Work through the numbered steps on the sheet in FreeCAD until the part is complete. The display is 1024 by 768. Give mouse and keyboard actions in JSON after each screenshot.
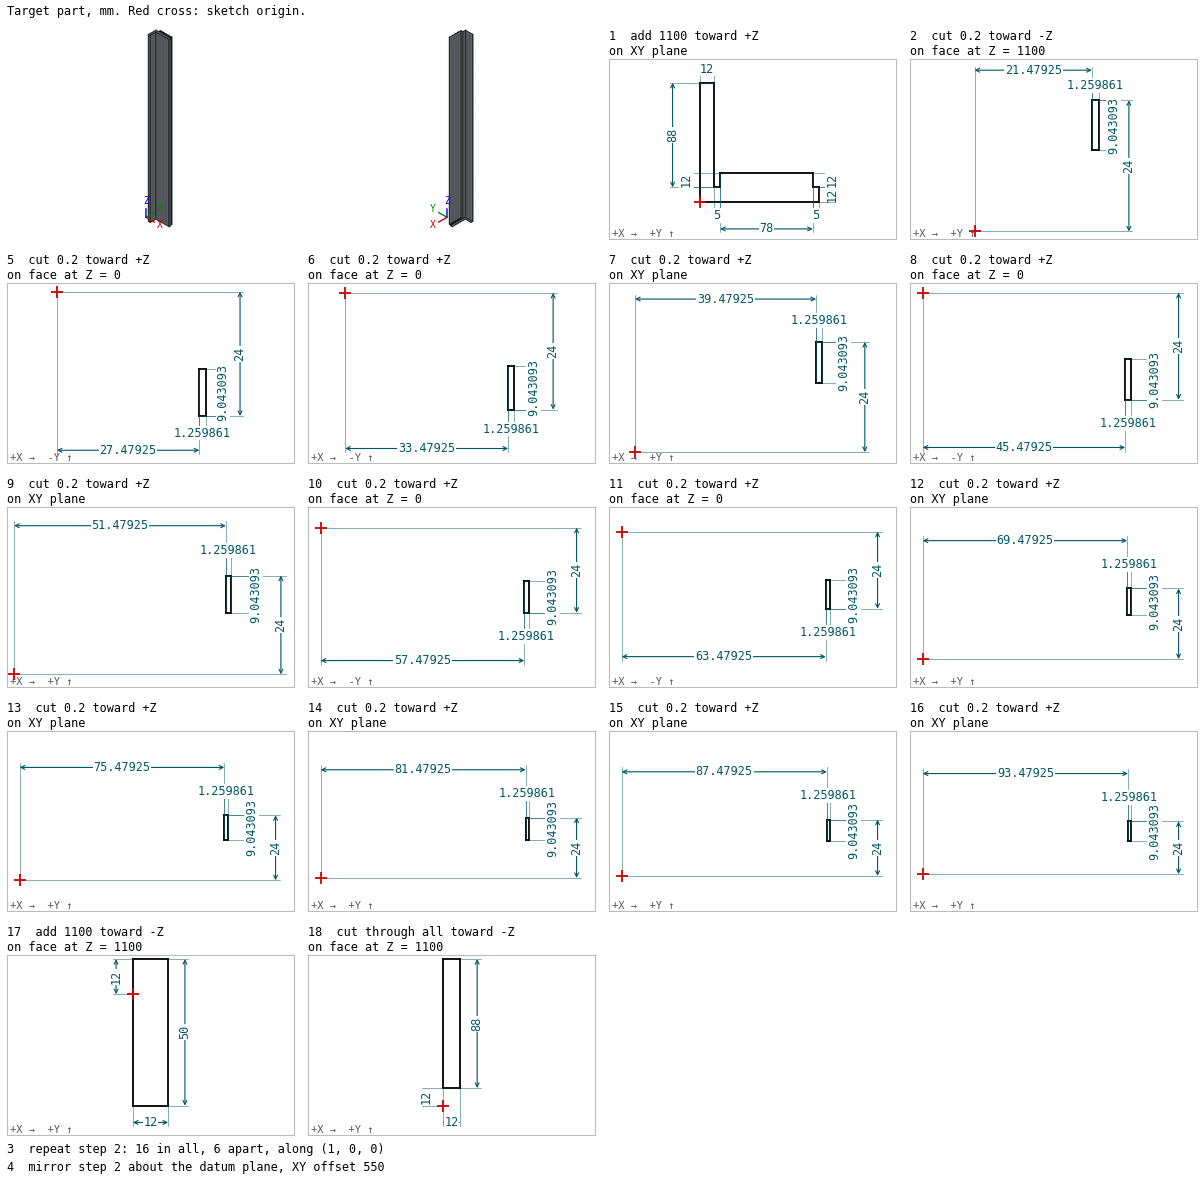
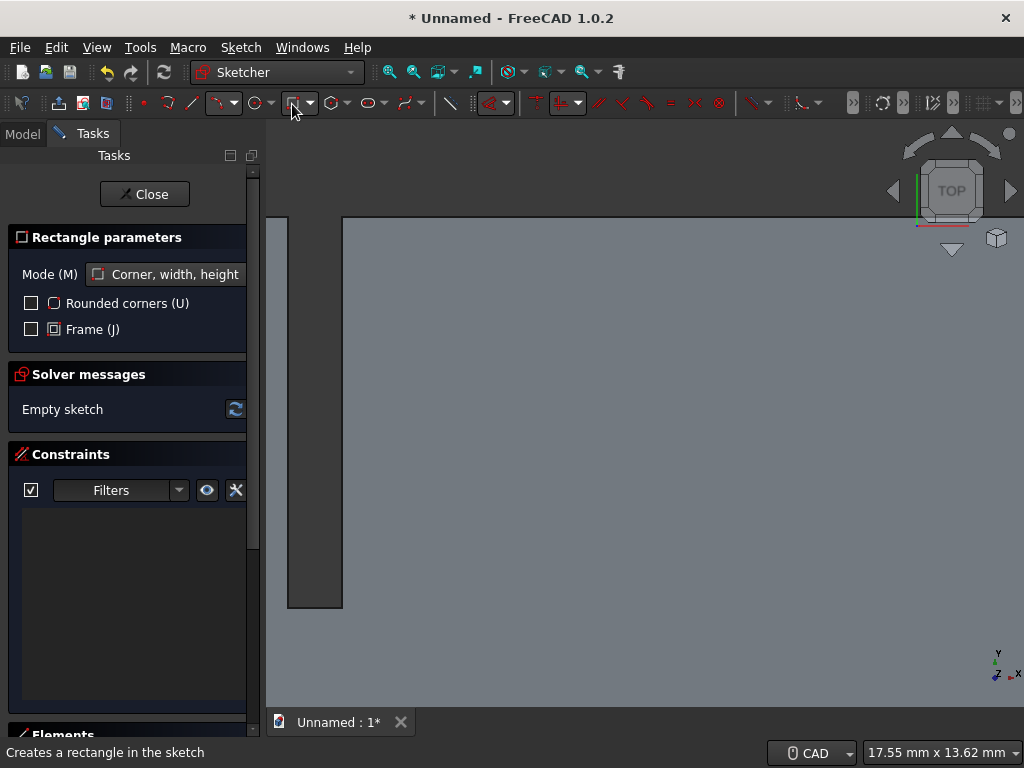
{"action": "left_click", "coordinate": [547, 217]}
{"action": "mouse_move", "coordinate": [601, 608]}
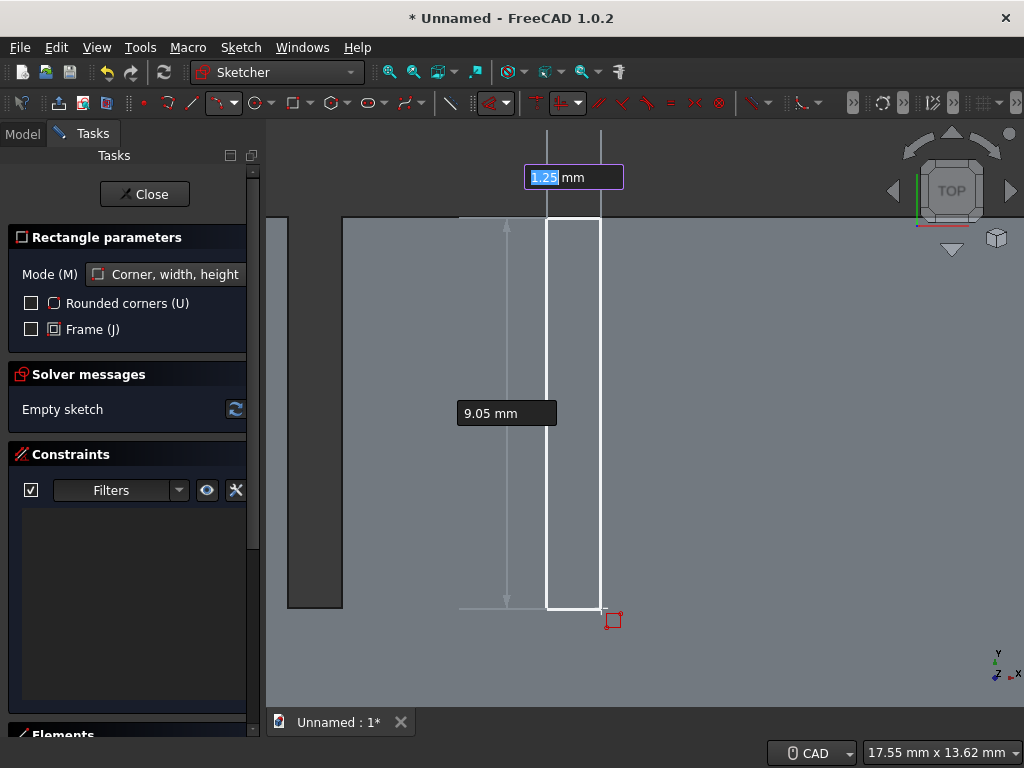
{"action": "type", "text": "1.259861"}
{"action": "key", "text": "Tab"}
{"action": "type", "text": "9.043093"}
{"action": "key", "text": "Return"}
{"action": "key", "text": "Escape"}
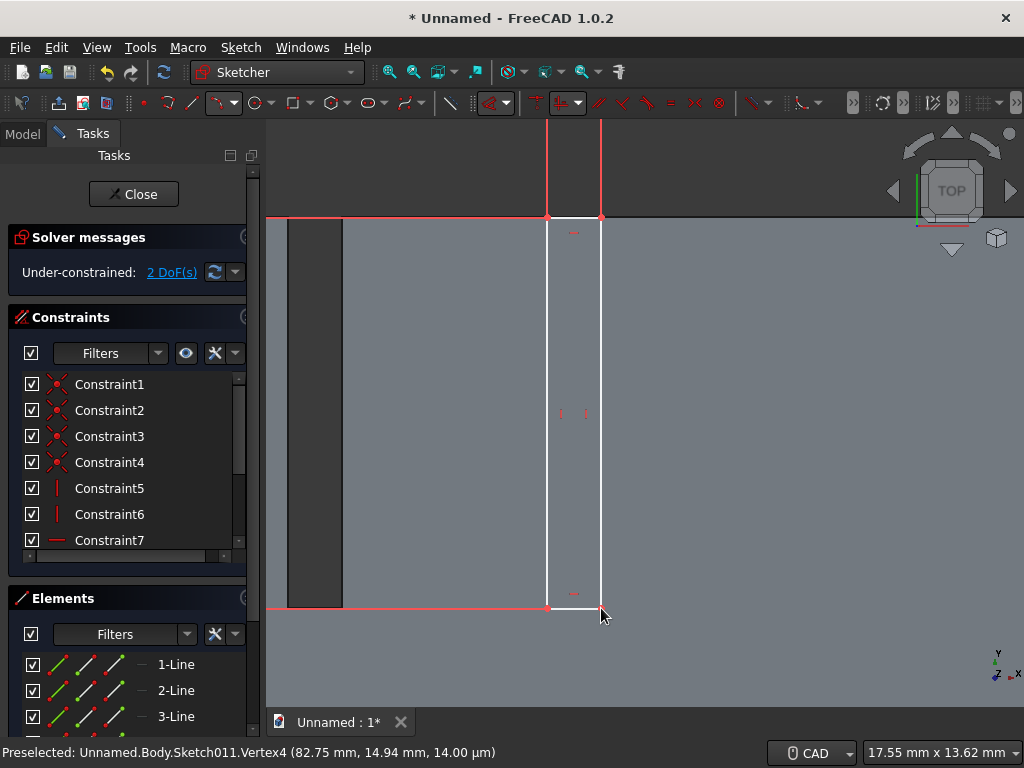
{"action": "left_click", "coordinate": [547, 218]}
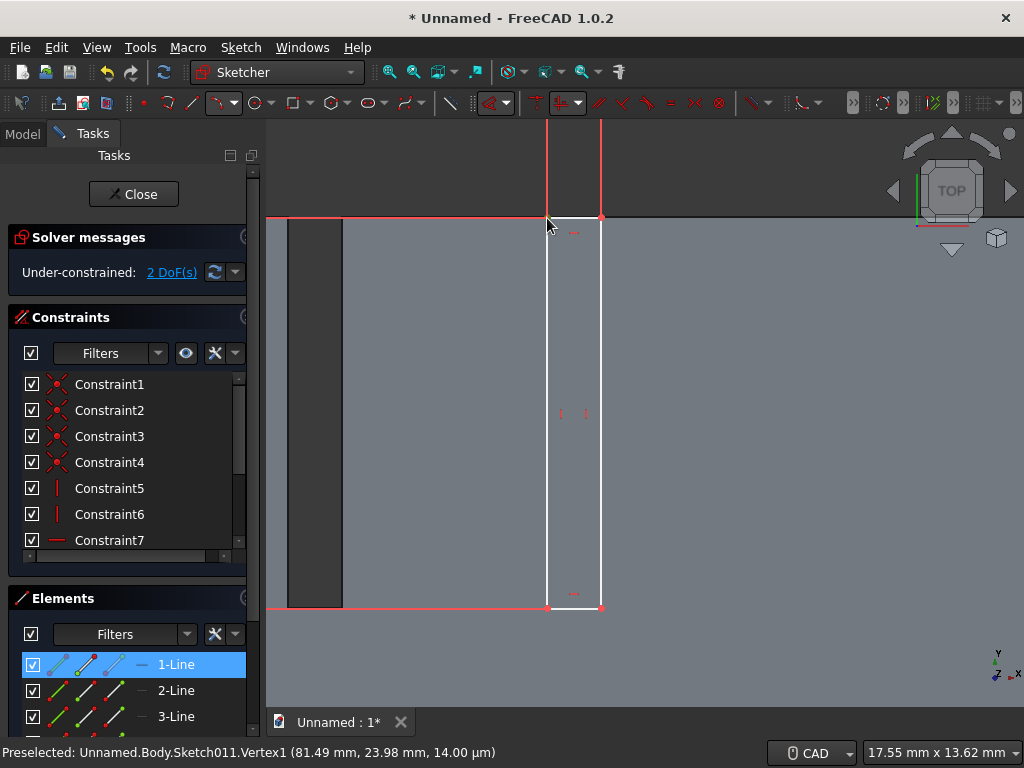
{"action": "left_click", "coordinate": [508, 104]}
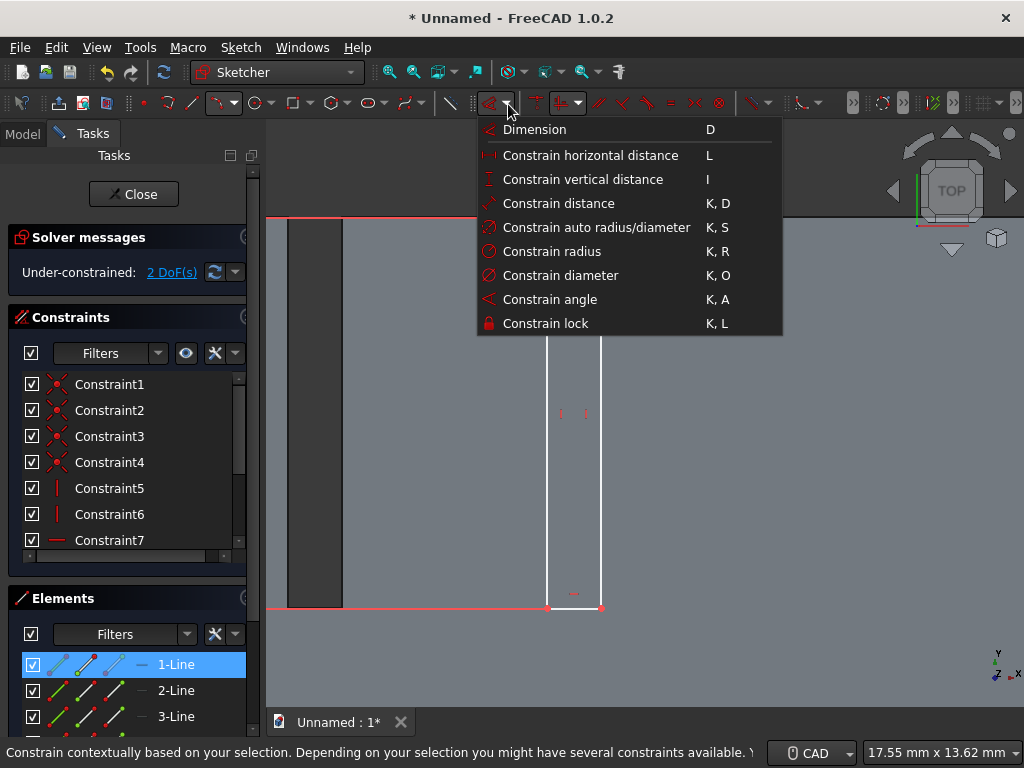
{"action": "left_click", "coordinate": [630, 179]}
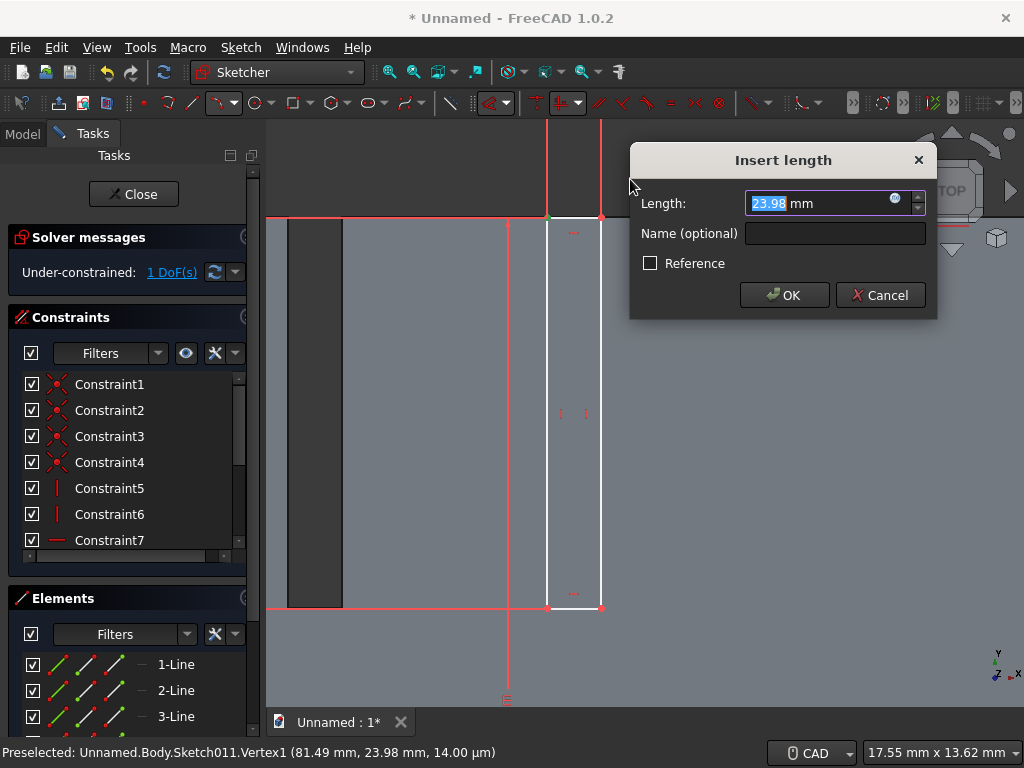
{"action": "type", "text": "24"}
{"action": "key", "text": "Return"}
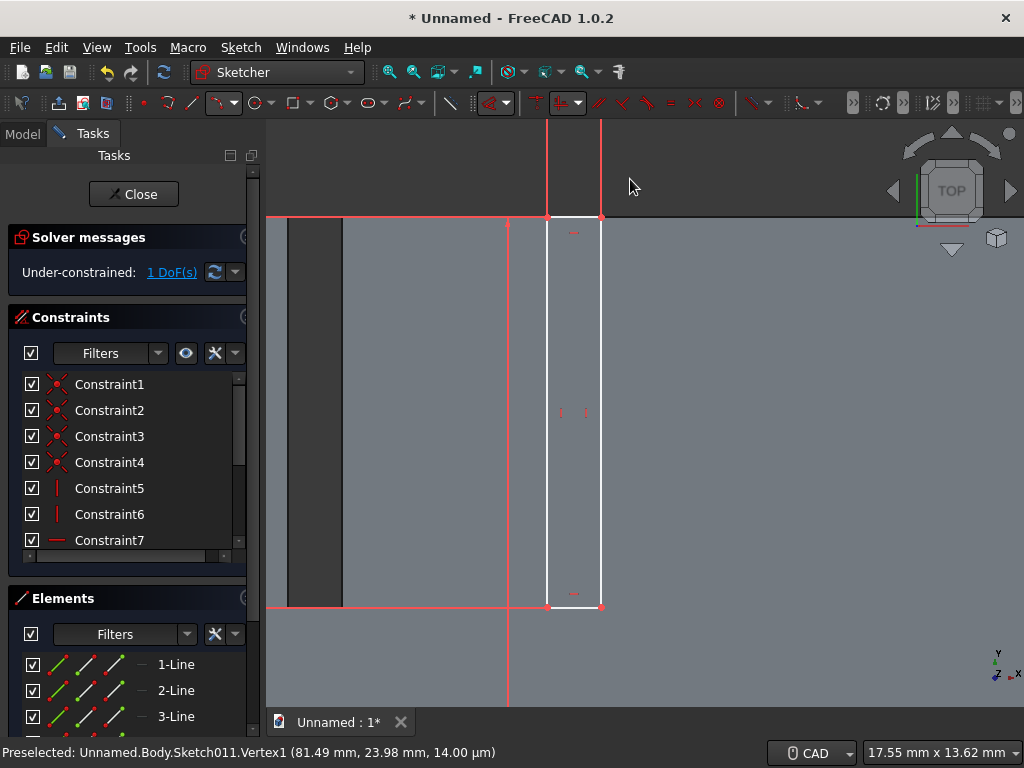
{"action": "left_click", "coordinate": [547, 217]}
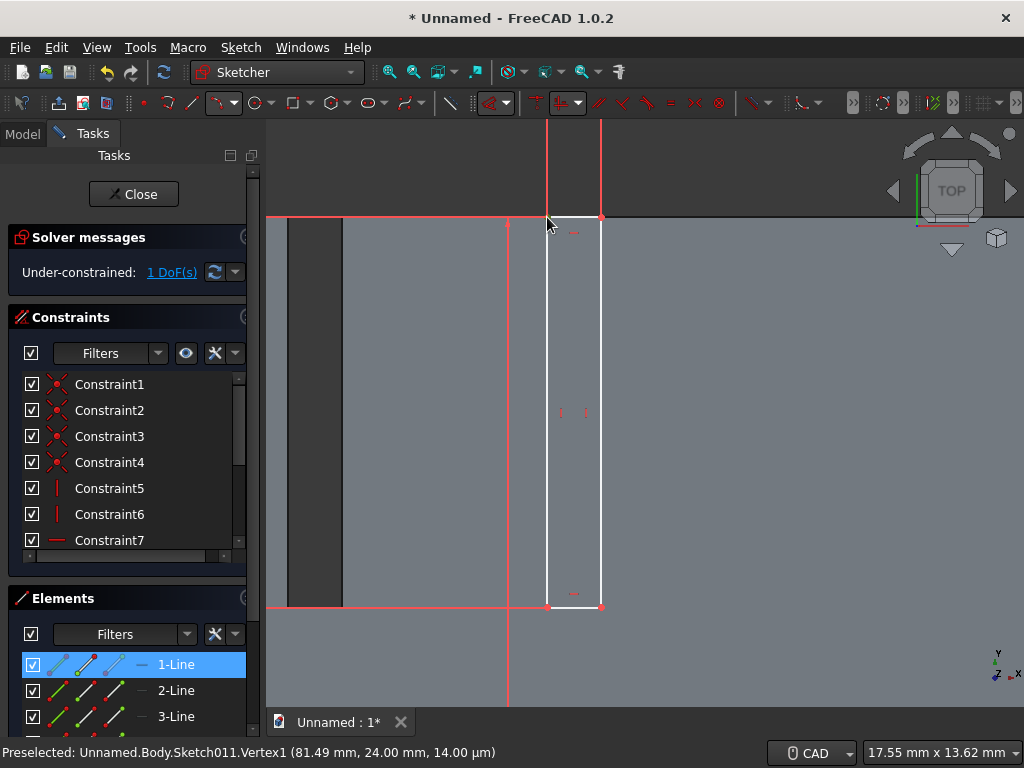
{"action": "key", "text": "l"}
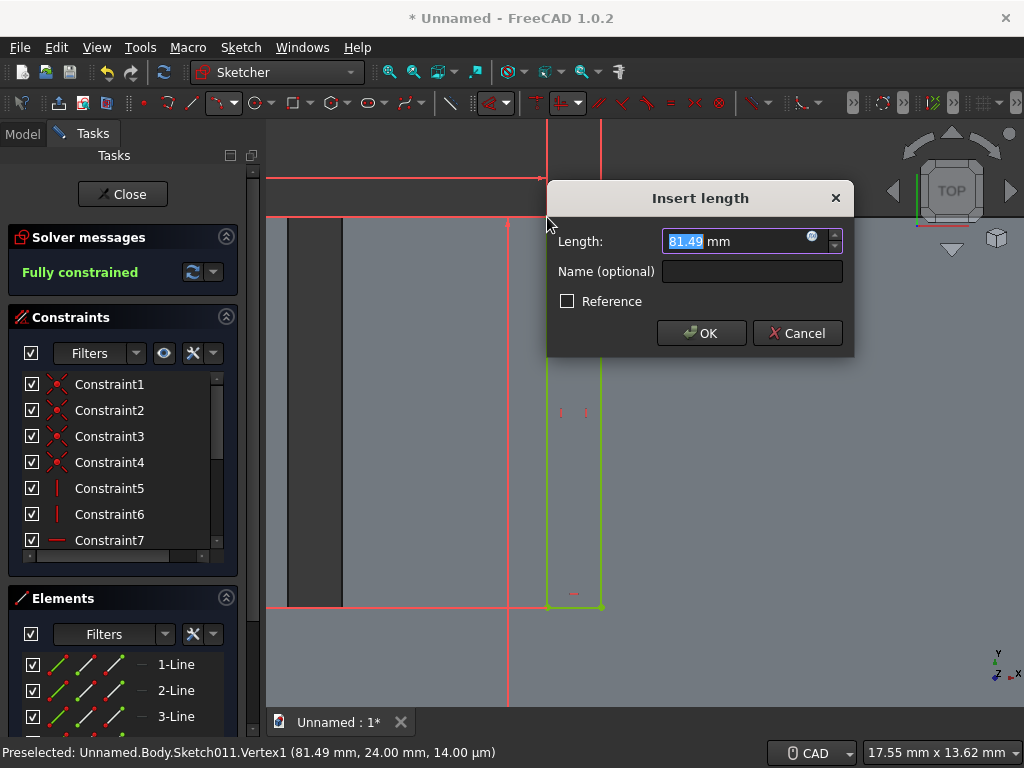
{"action": "type", "text": "81.47925"}
{"action": "key", "text": "Return"}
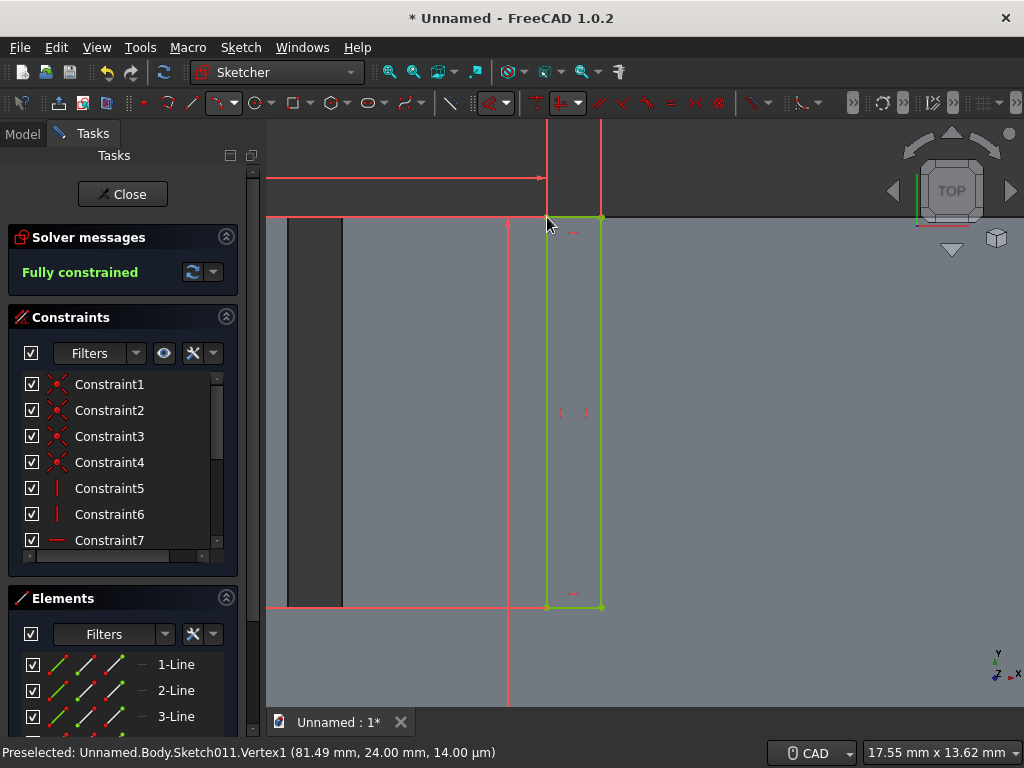
{"action": "left_click", "coordinate": [123, 194]}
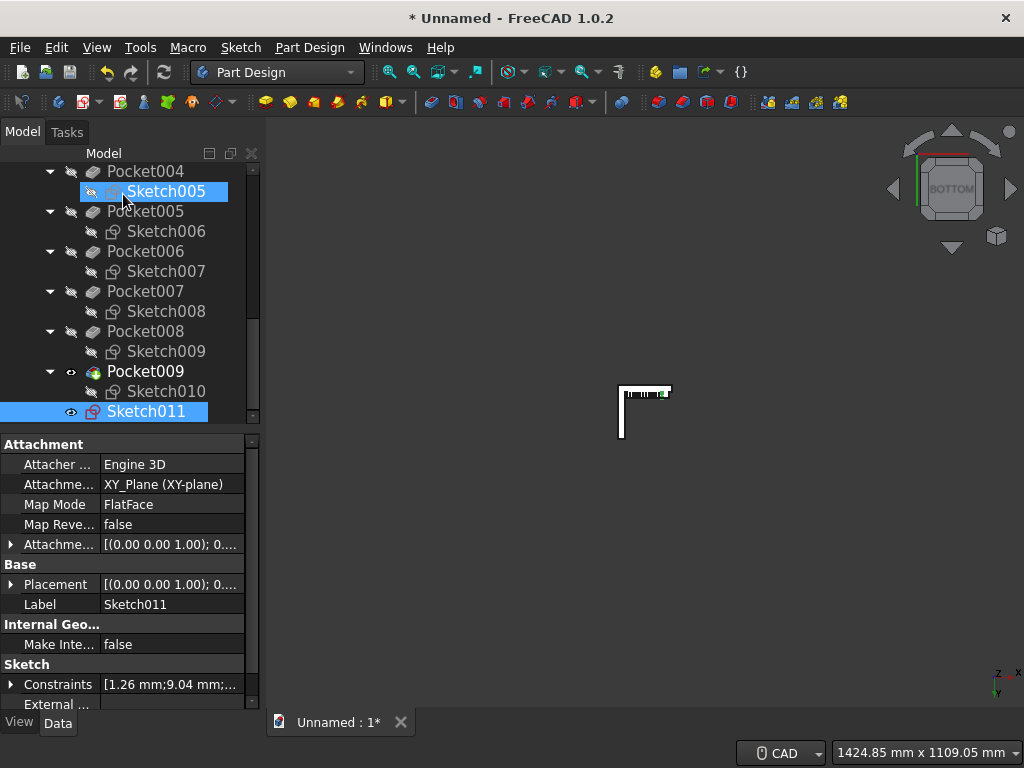
{"action": "left_click", "coordinate": [432, 102]}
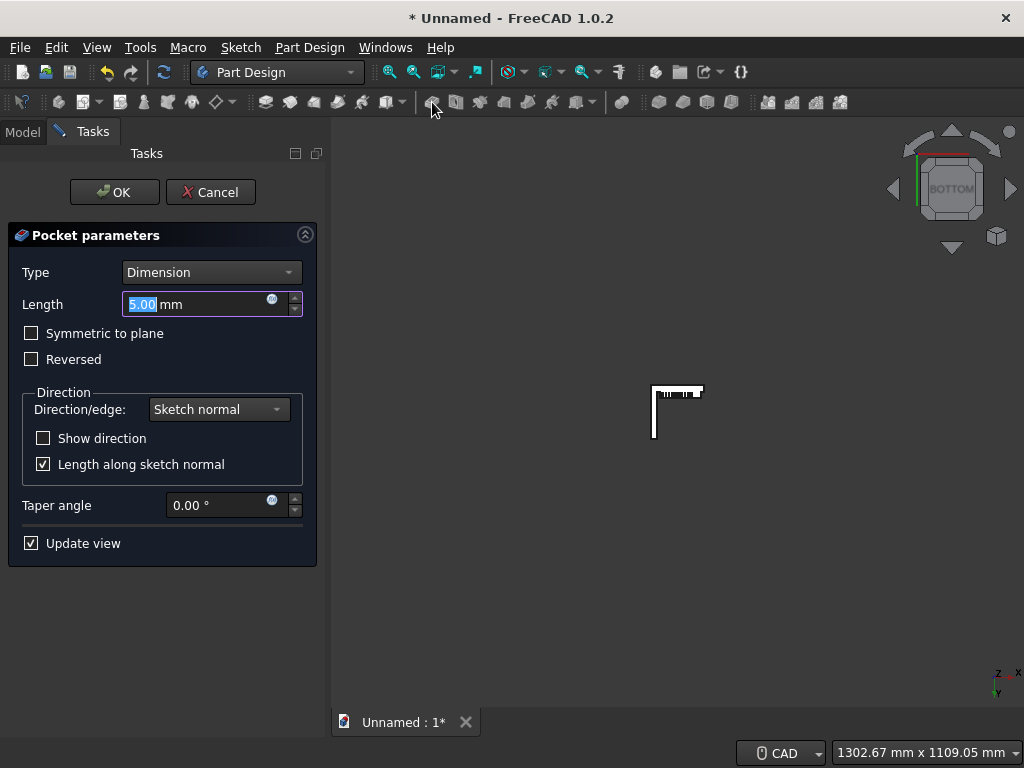
{"action": "type", "text": "0.2"}
{"action": "key", "text": "Tab"}